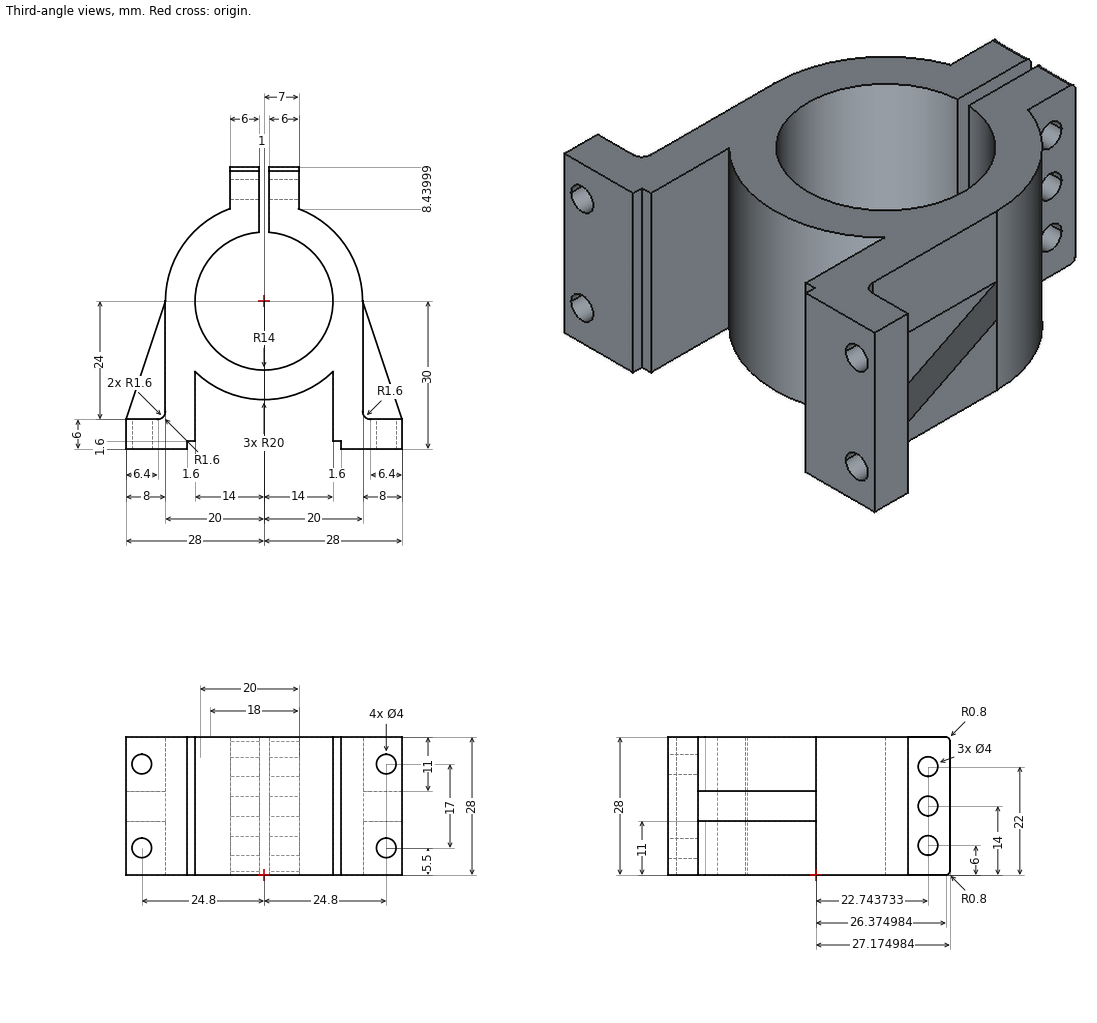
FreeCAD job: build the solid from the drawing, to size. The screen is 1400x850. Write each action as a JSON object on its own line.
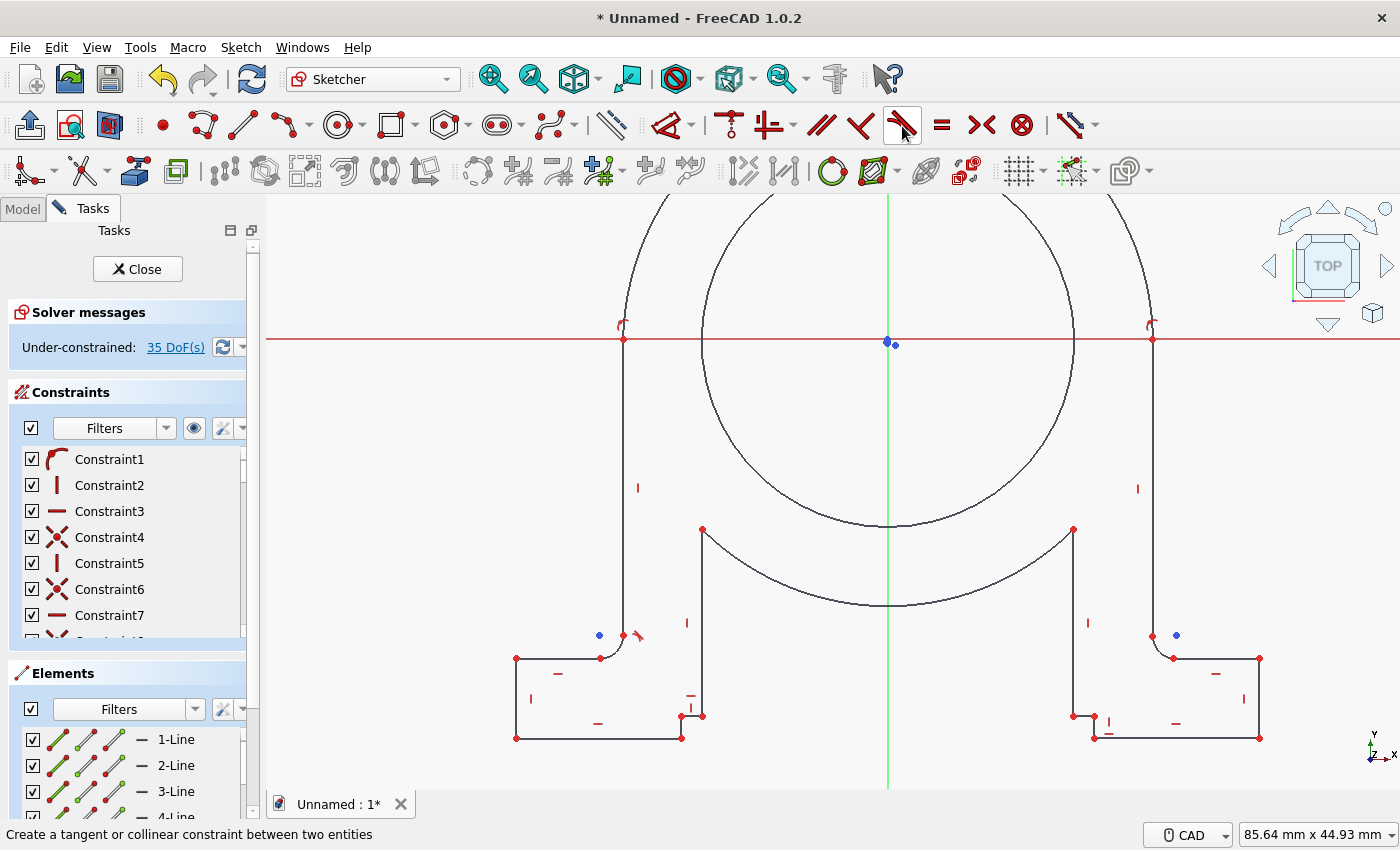
{"action": "left_click", "coordinate": [623, 428]}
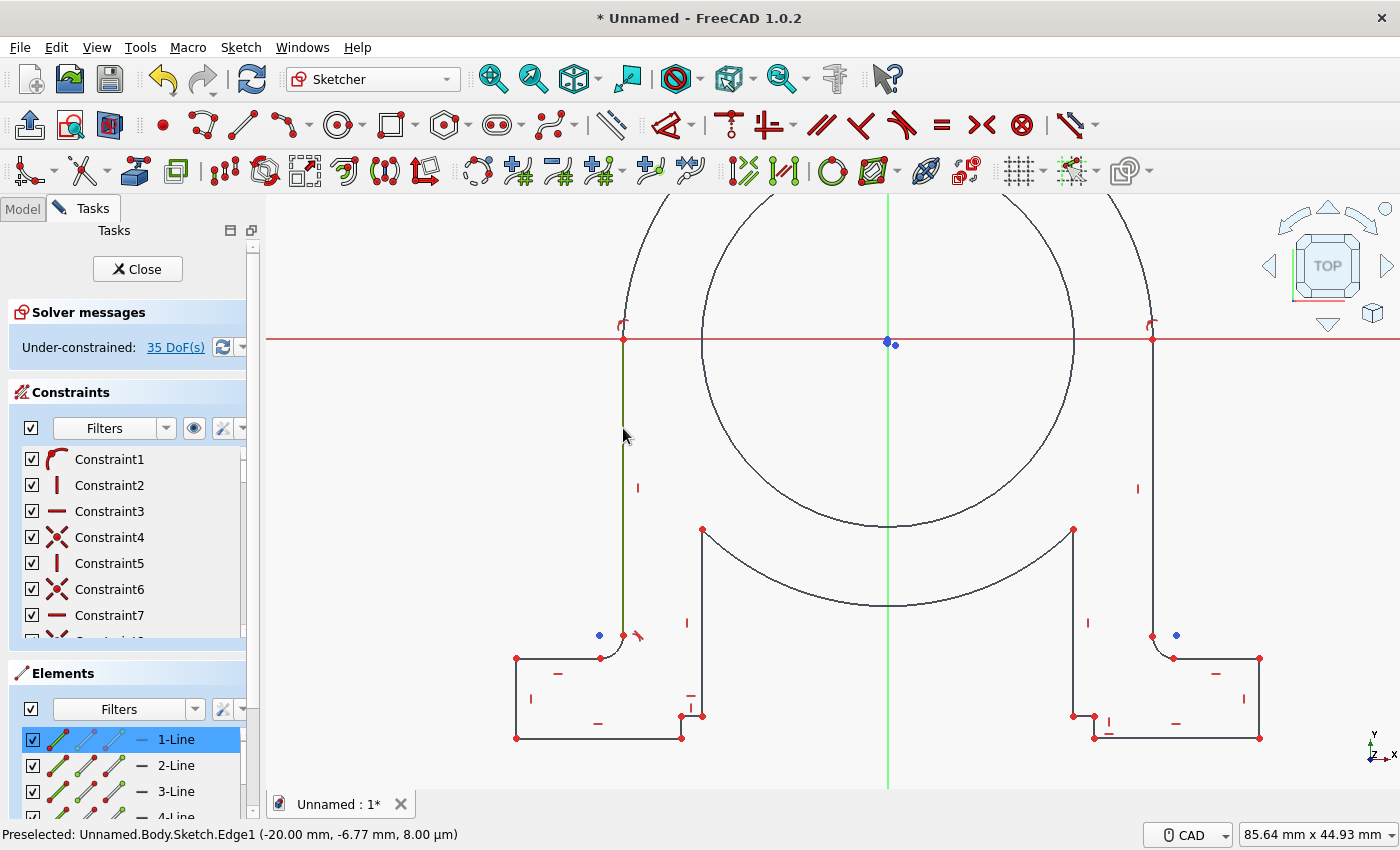
{"action": "left_click", "coordinate": [642, 246]}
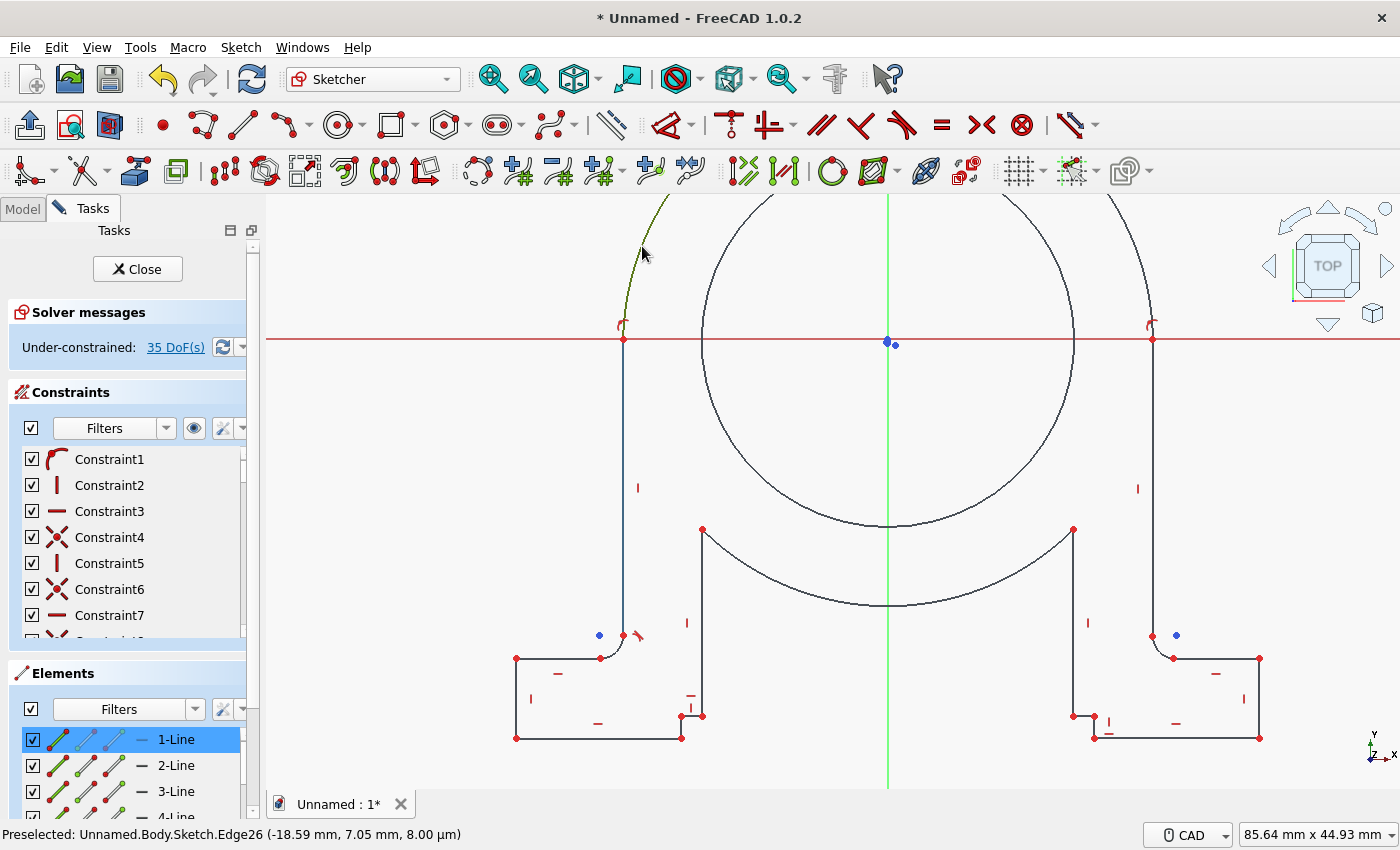
{"action": "left_click", "coordinate": [902, 126]}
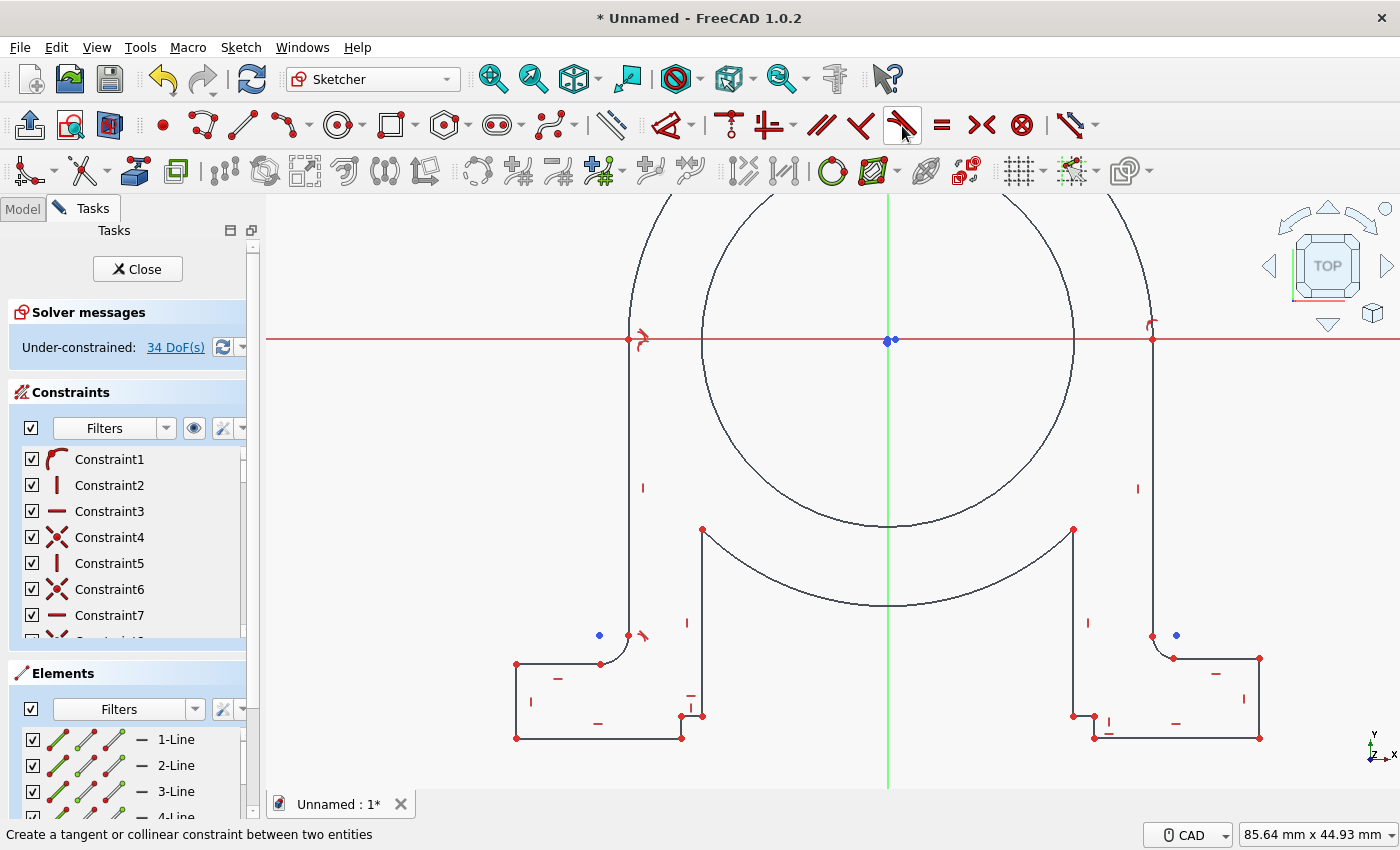
{"action": "left_click", "coordinate": [576, 664]}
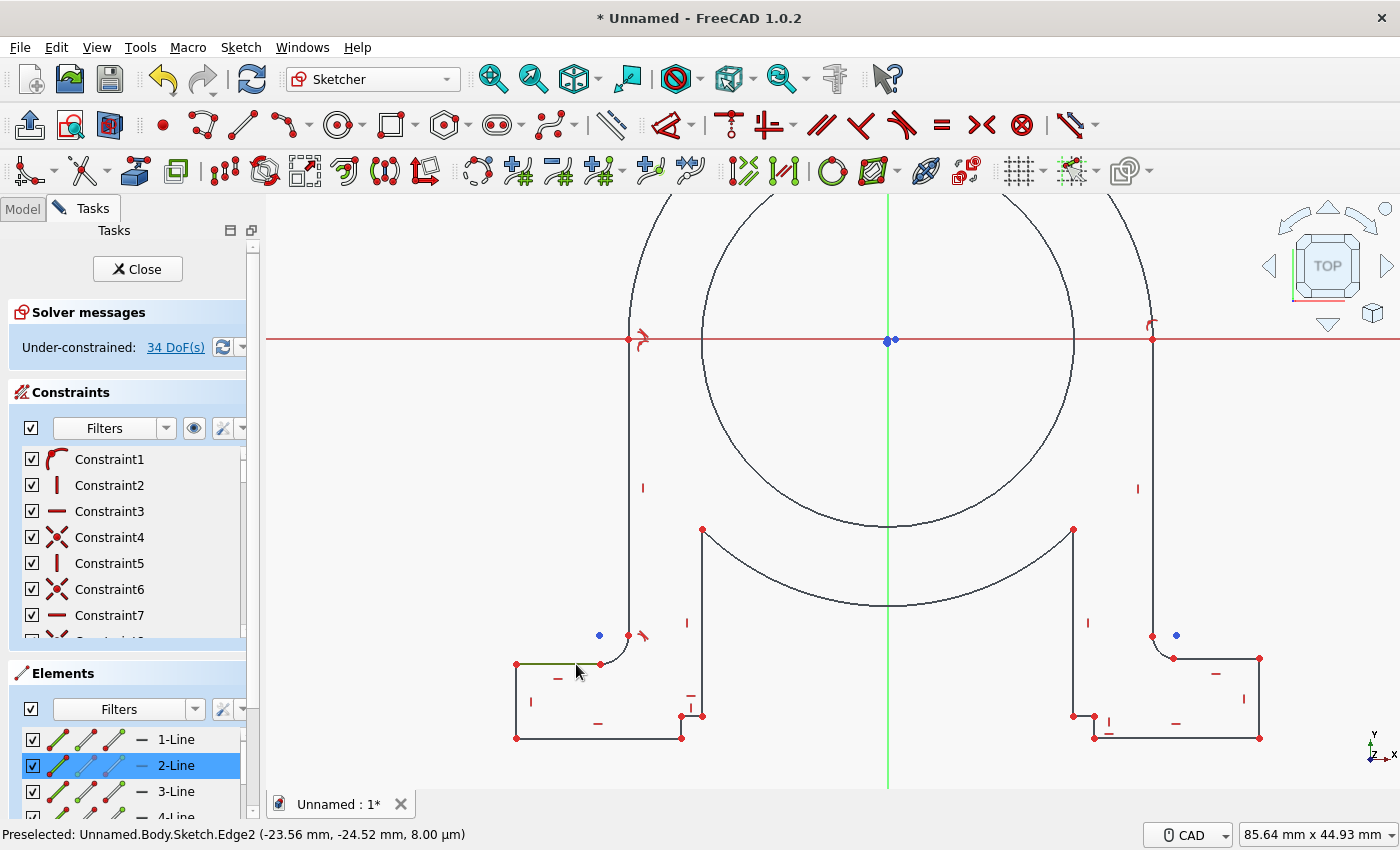
{"action": "left_click", "coordinate": [614, 661]}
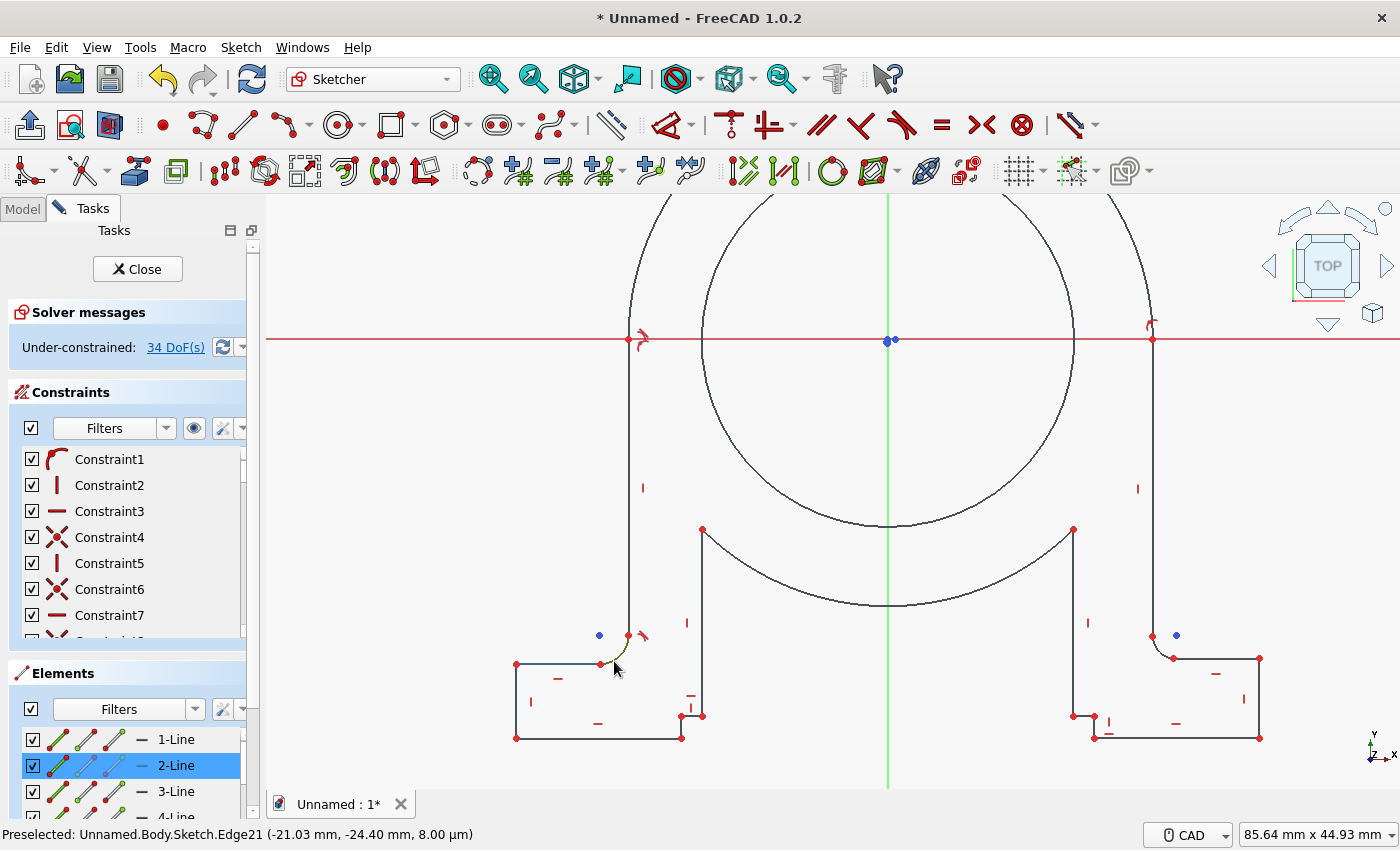
{"action": "left_click", "coordinate": [902, 126]}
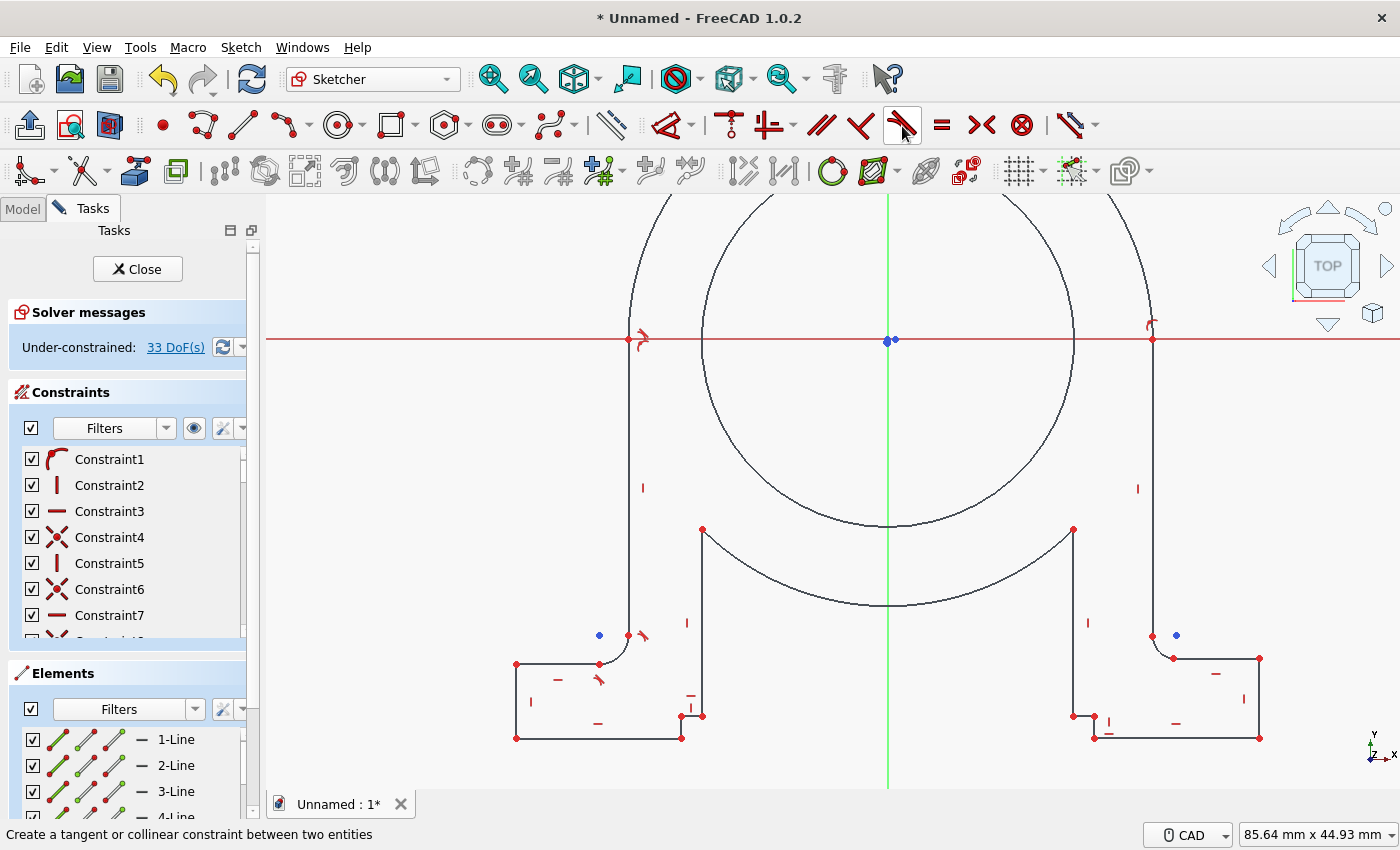
{"action": "left_click", "coordinate": [1234, 659]}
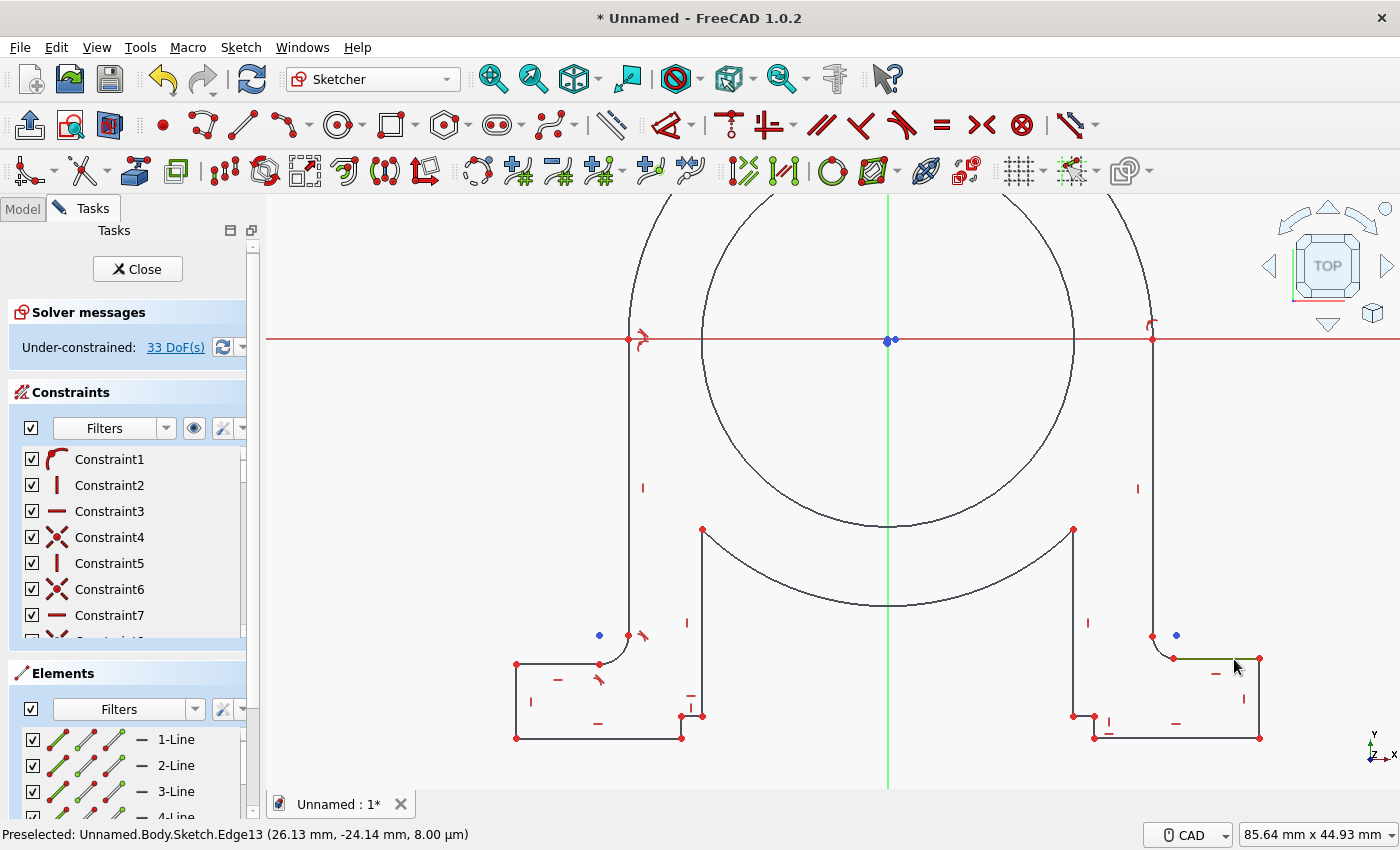
{"action": "scroll", "coordinate": [1156, 646], "scroll_direction": "up", "scroll_amount": 2}